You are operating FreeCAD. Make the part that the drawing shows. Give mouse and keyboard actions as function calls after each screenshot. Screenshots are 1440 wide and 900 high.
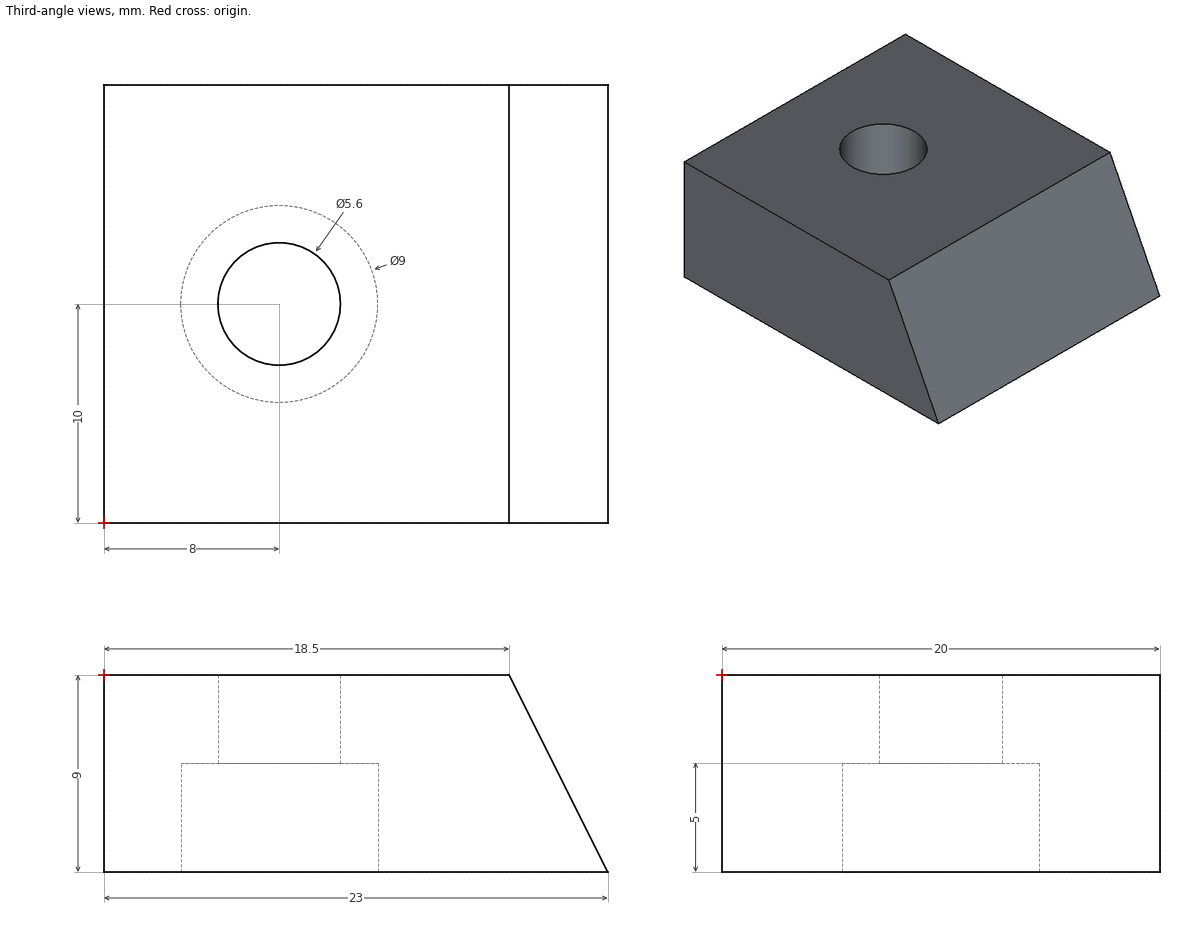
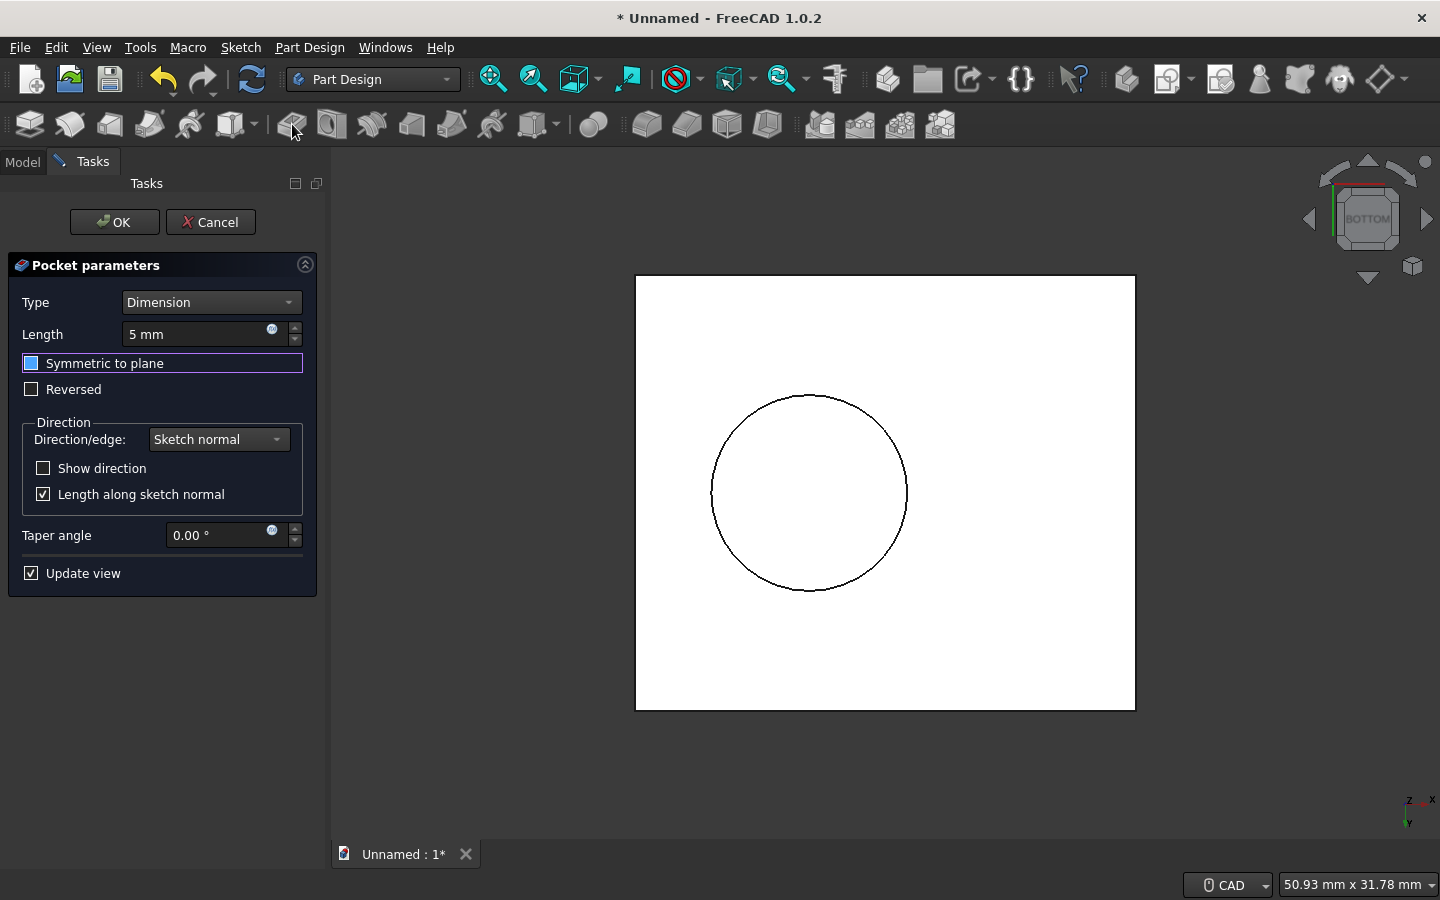
click(115, 222)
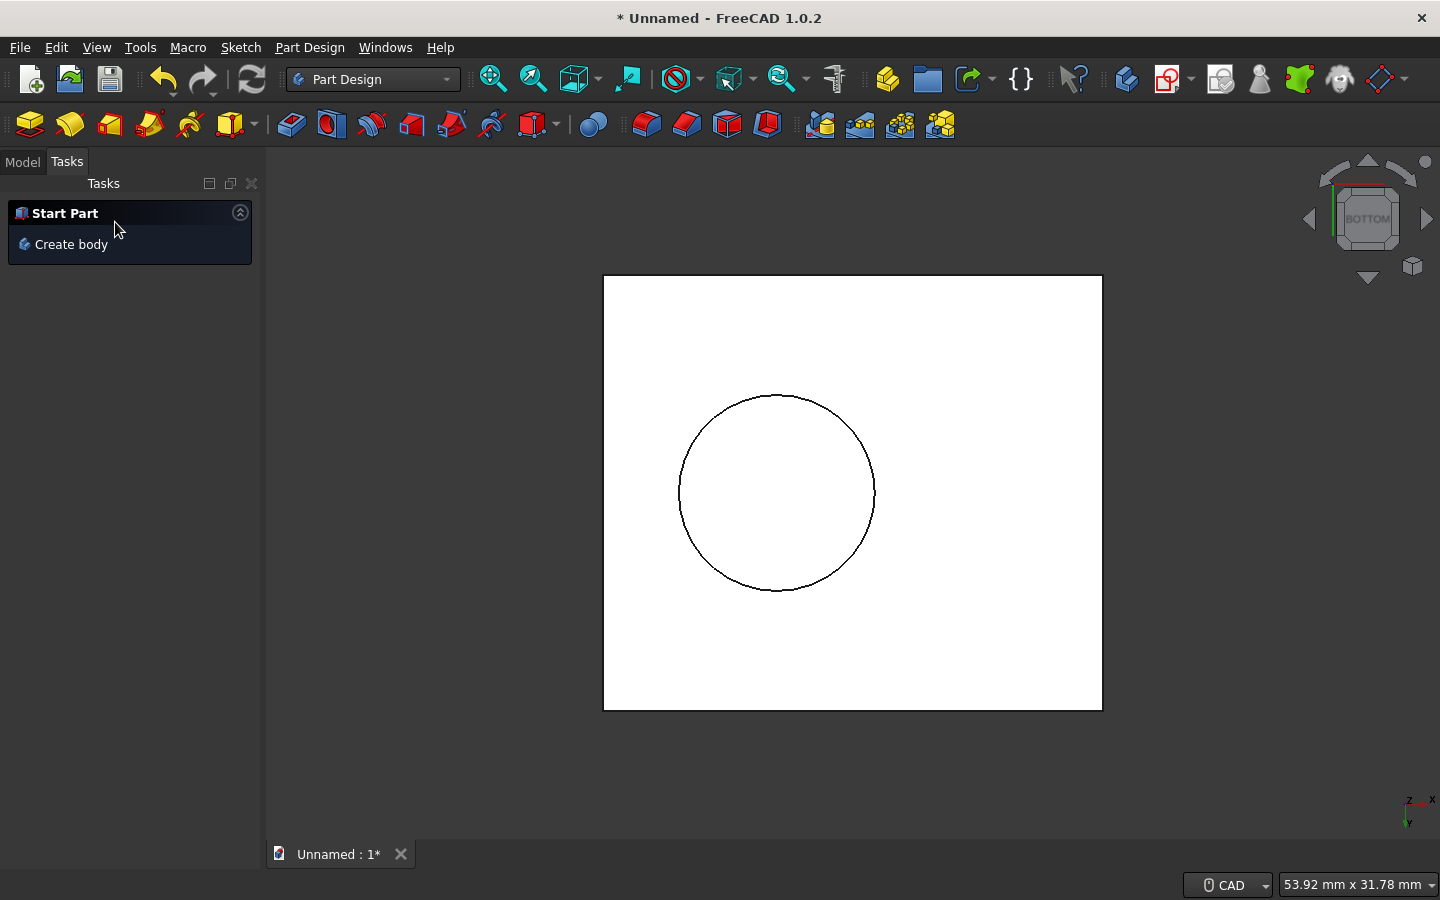
click(777, 492)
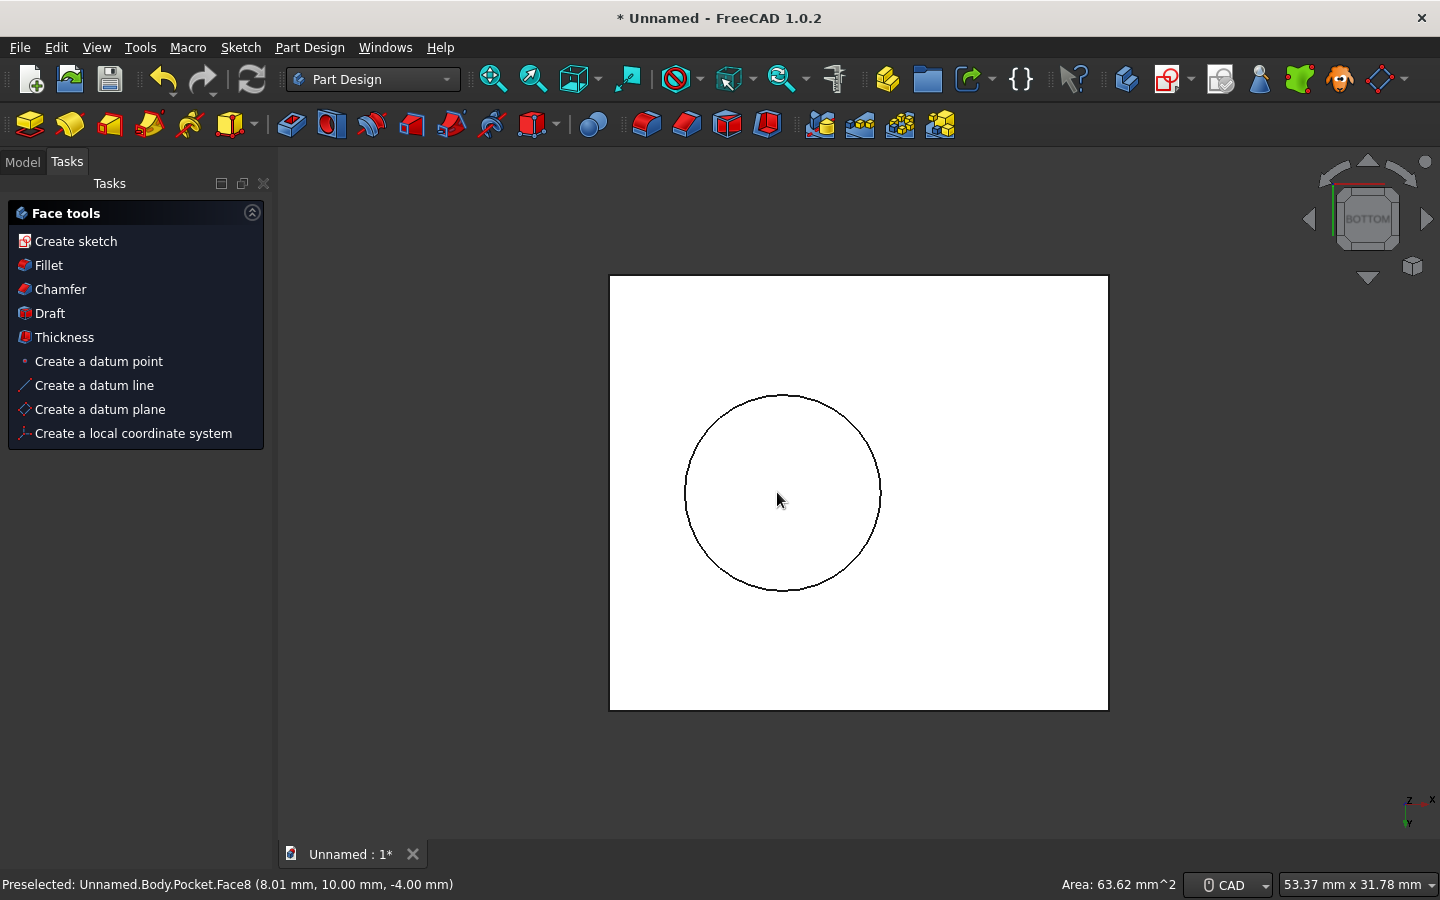
click(1168, 80)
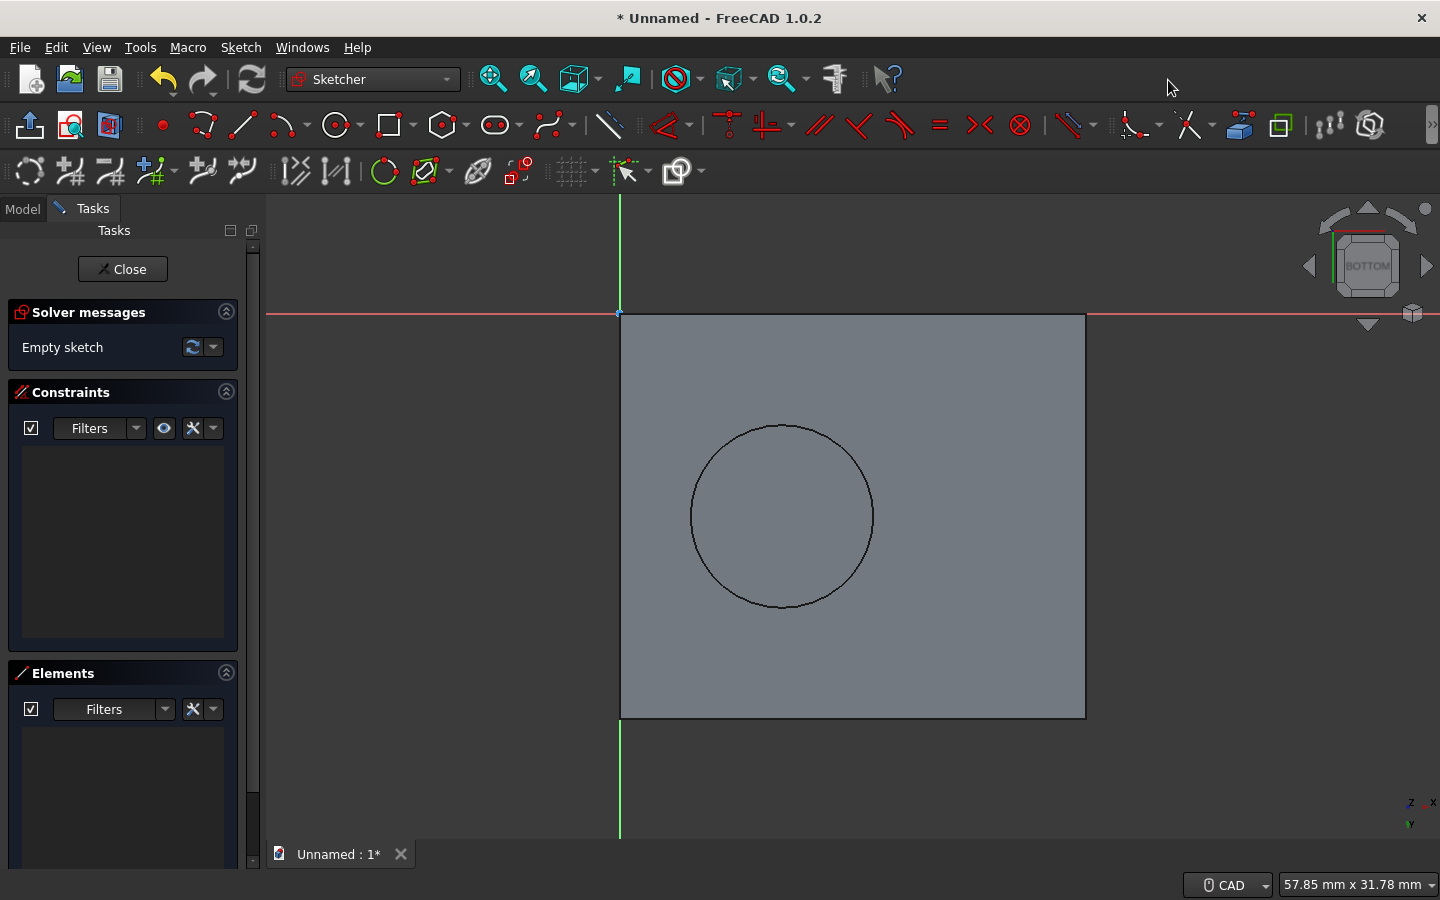
click(110, 126)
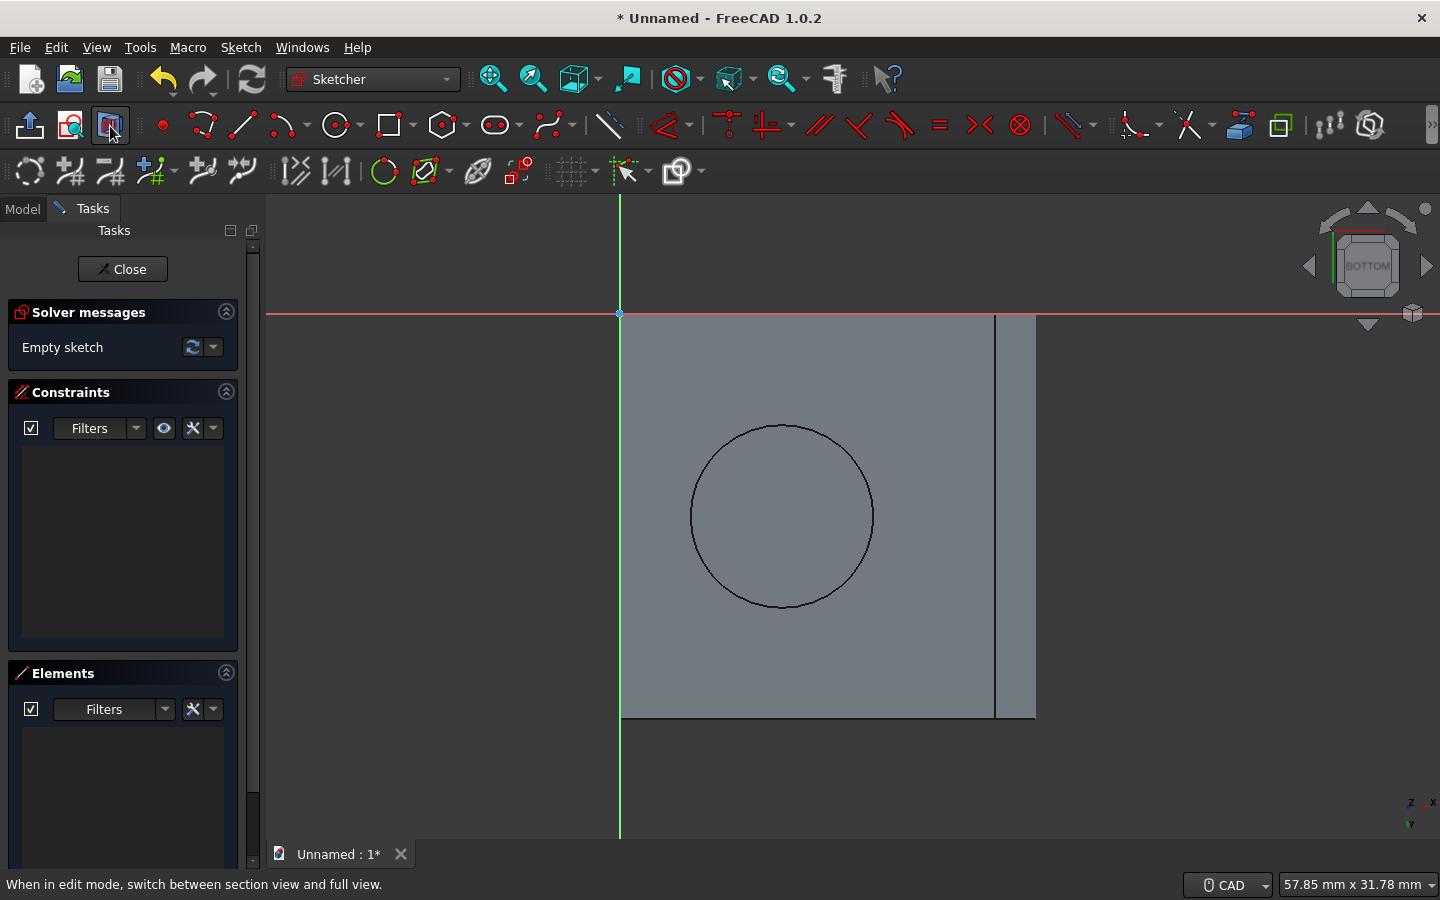
scroll(617, 295, up, 2)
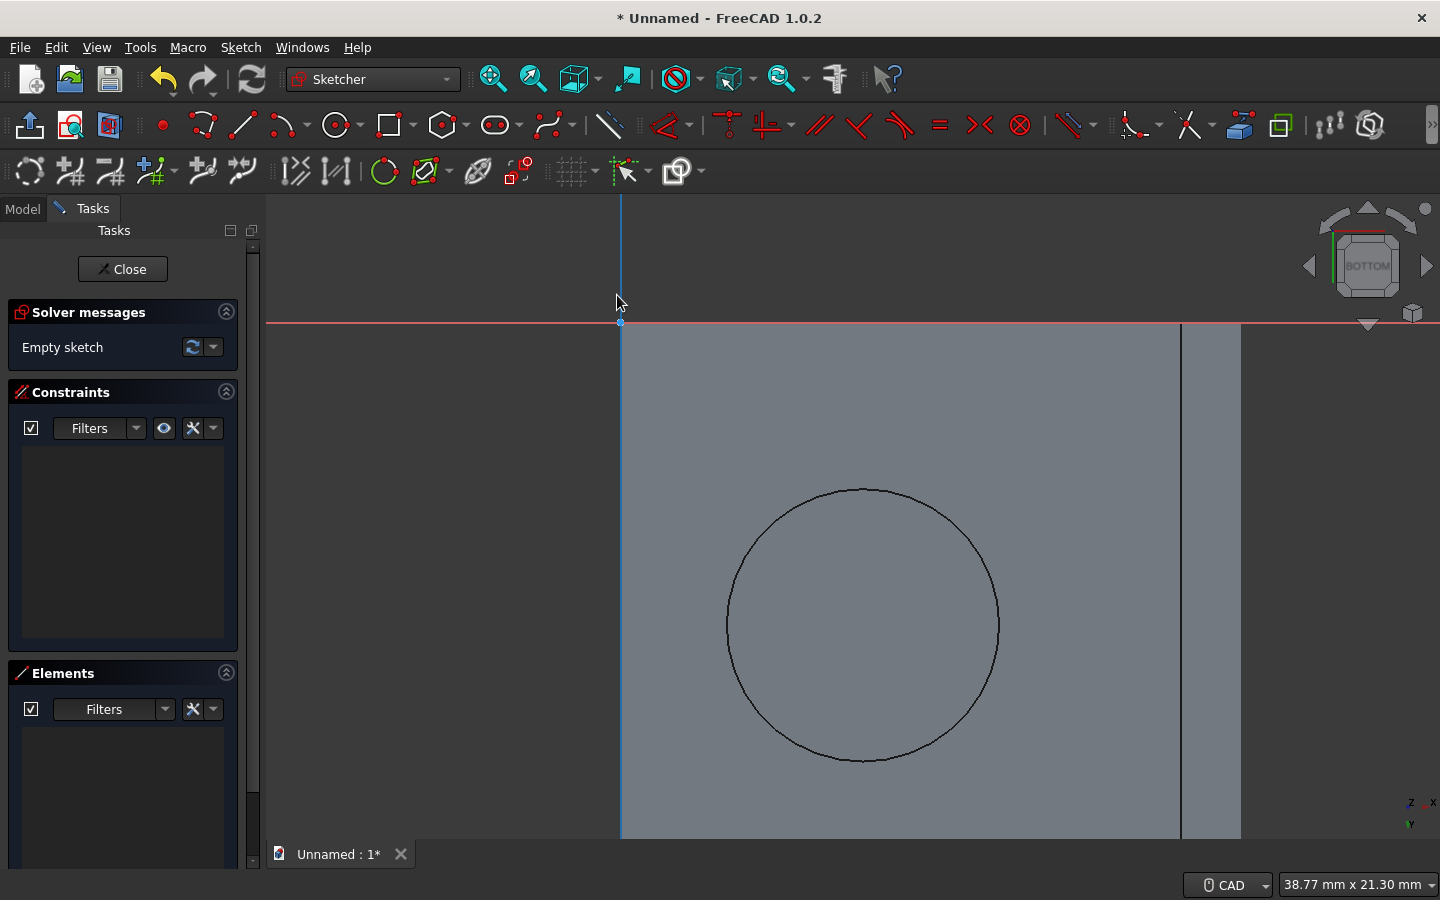
click(336, 126)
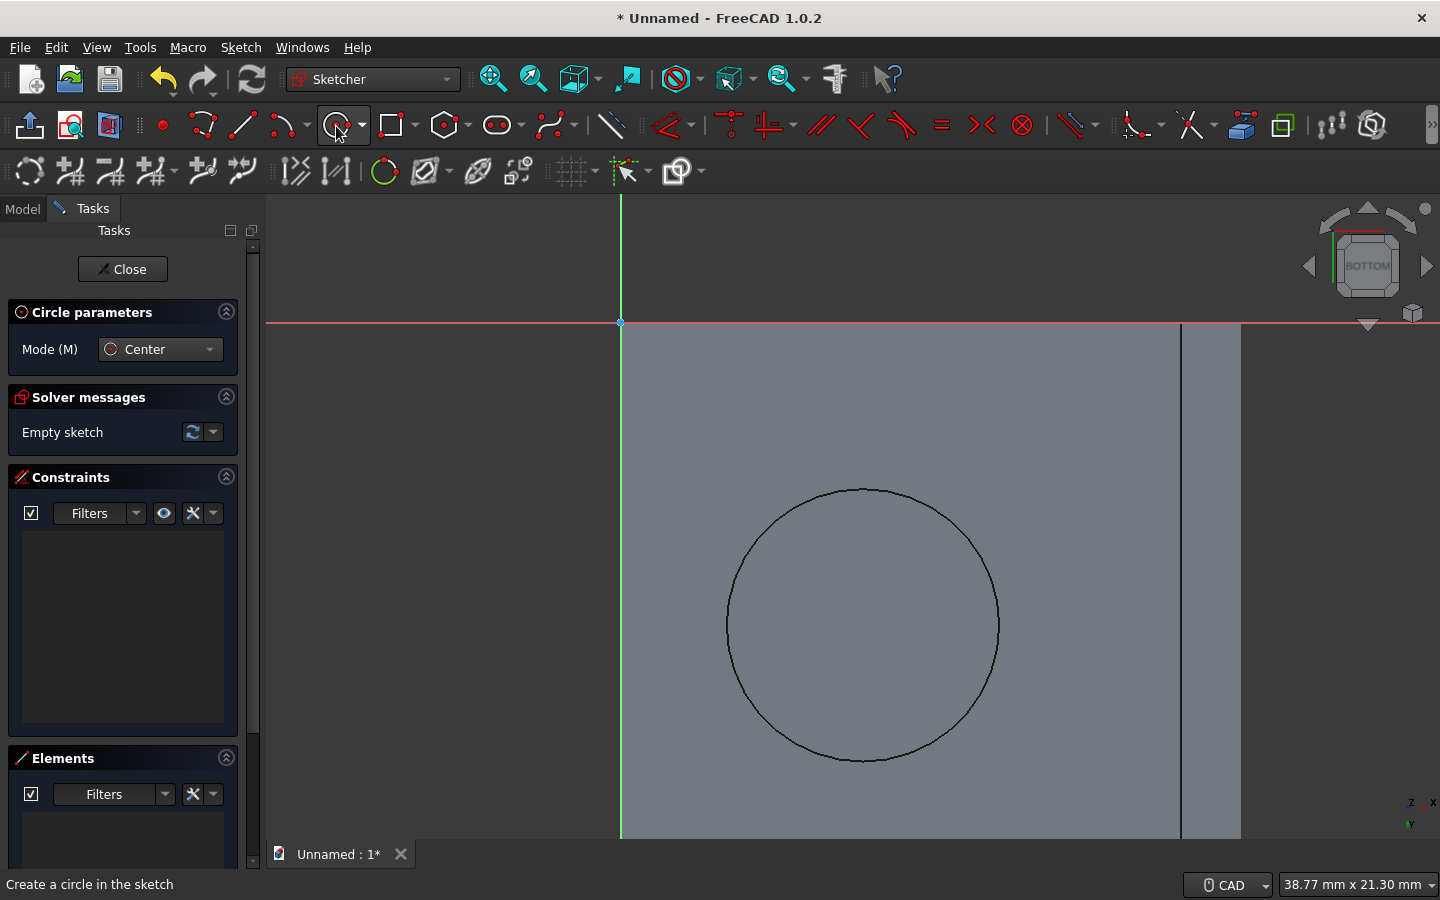
click(863, 625)
move(923, 565)